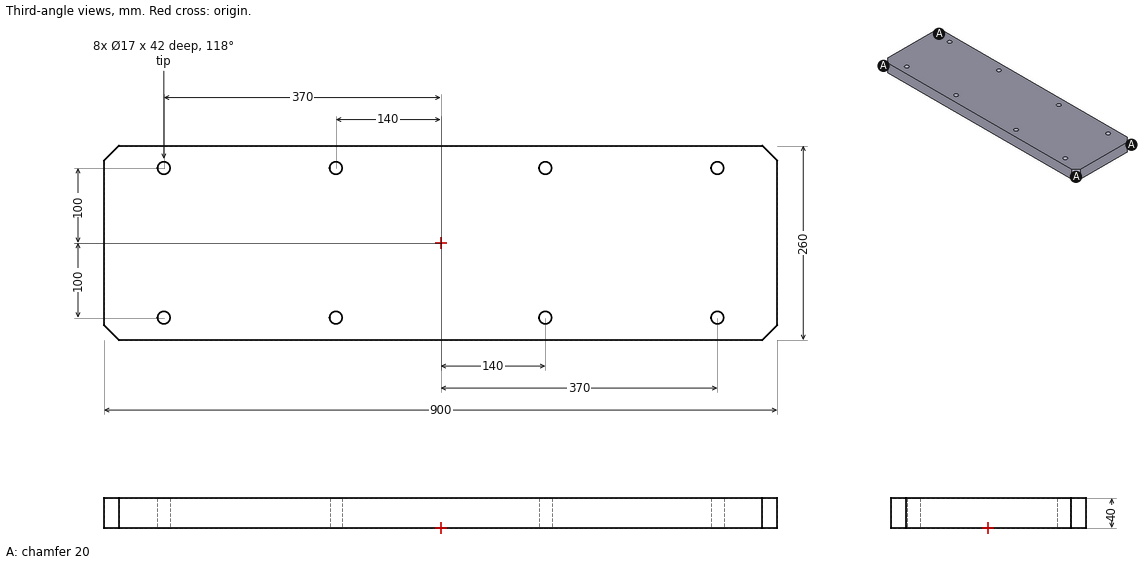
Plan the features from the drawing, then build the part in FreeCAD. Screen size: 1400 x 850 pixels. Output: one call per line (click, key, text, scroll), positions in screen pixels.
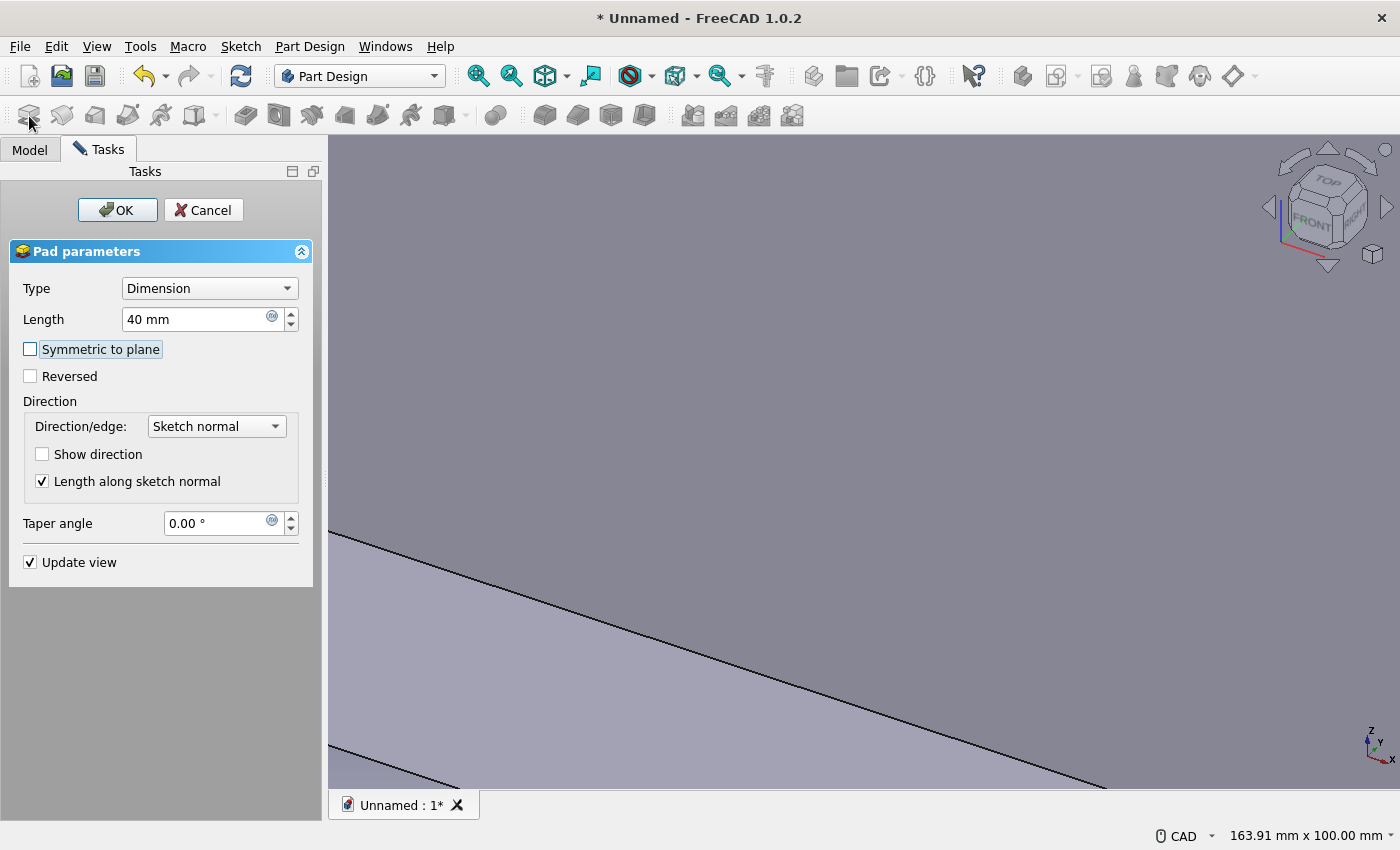
click(118, 210)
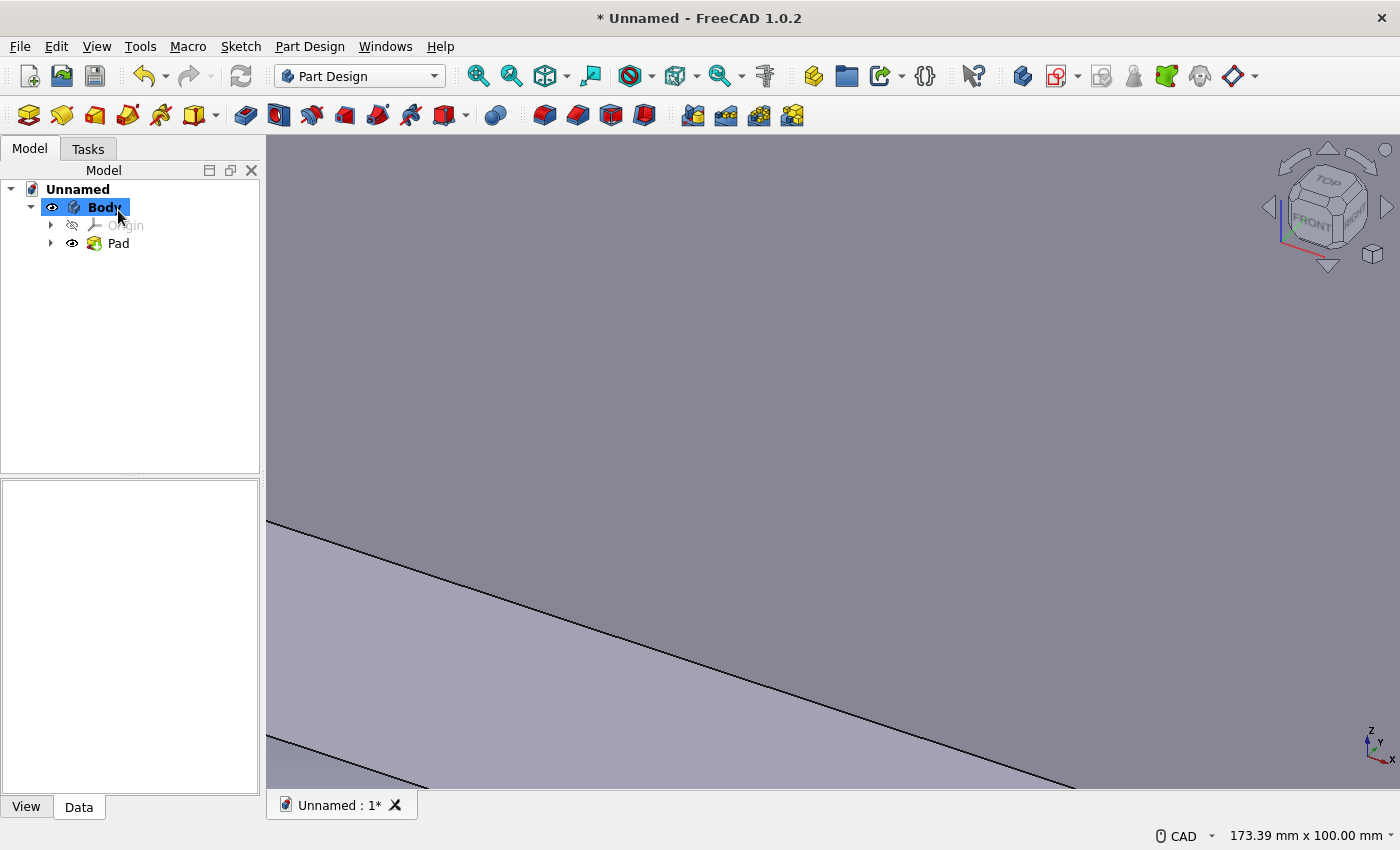
click(479, 76)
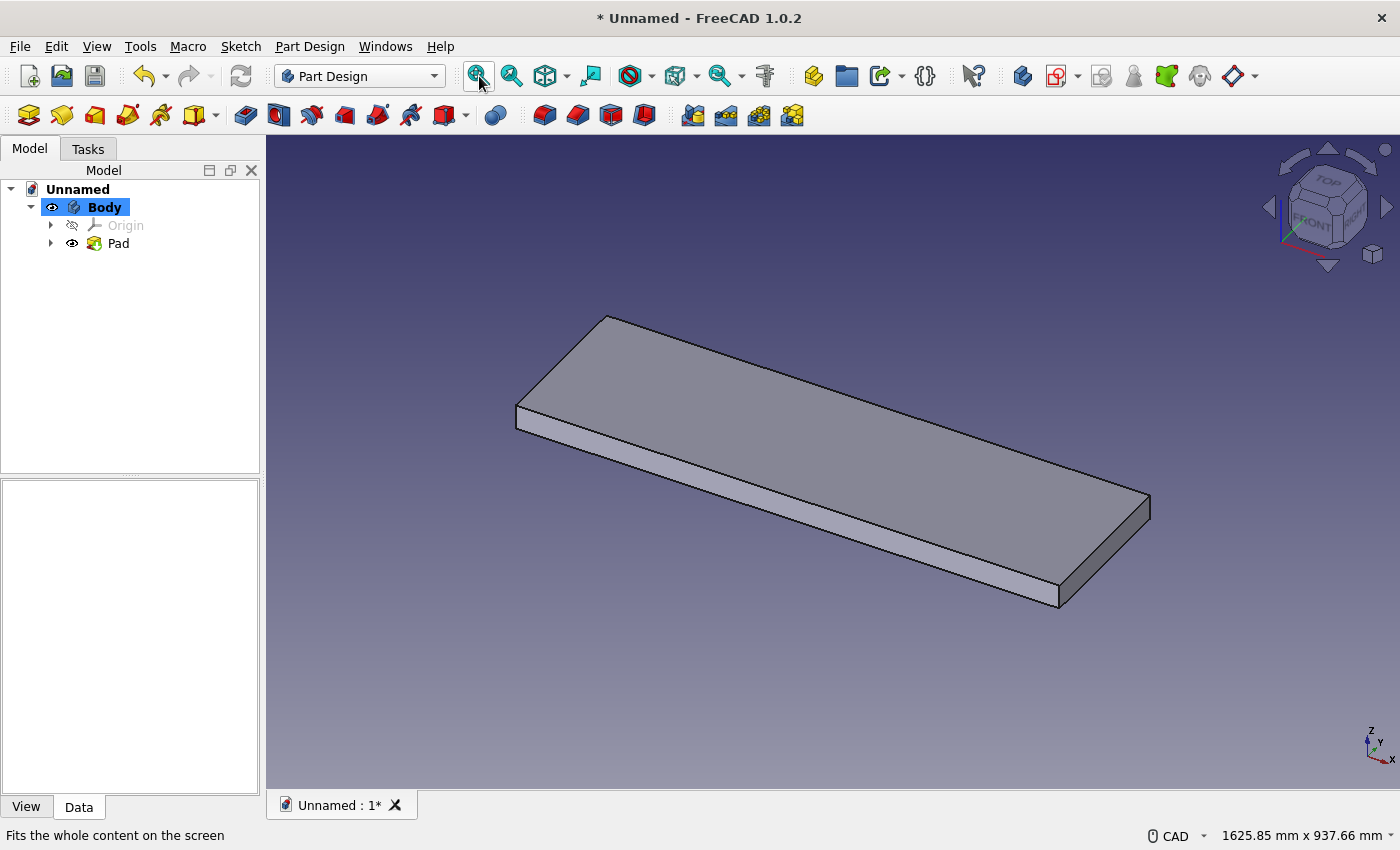
click(988, 501)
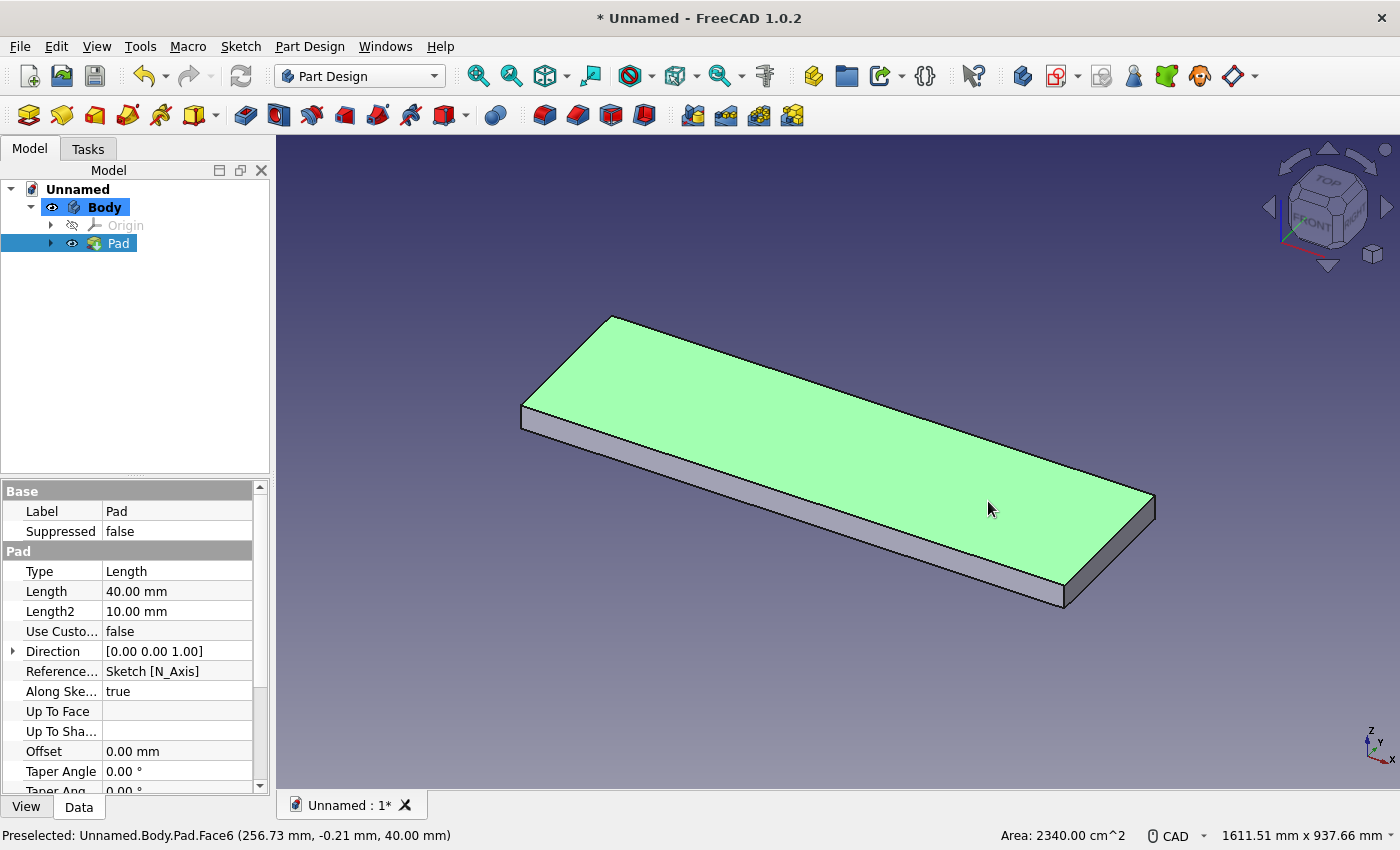
click(1056, 76)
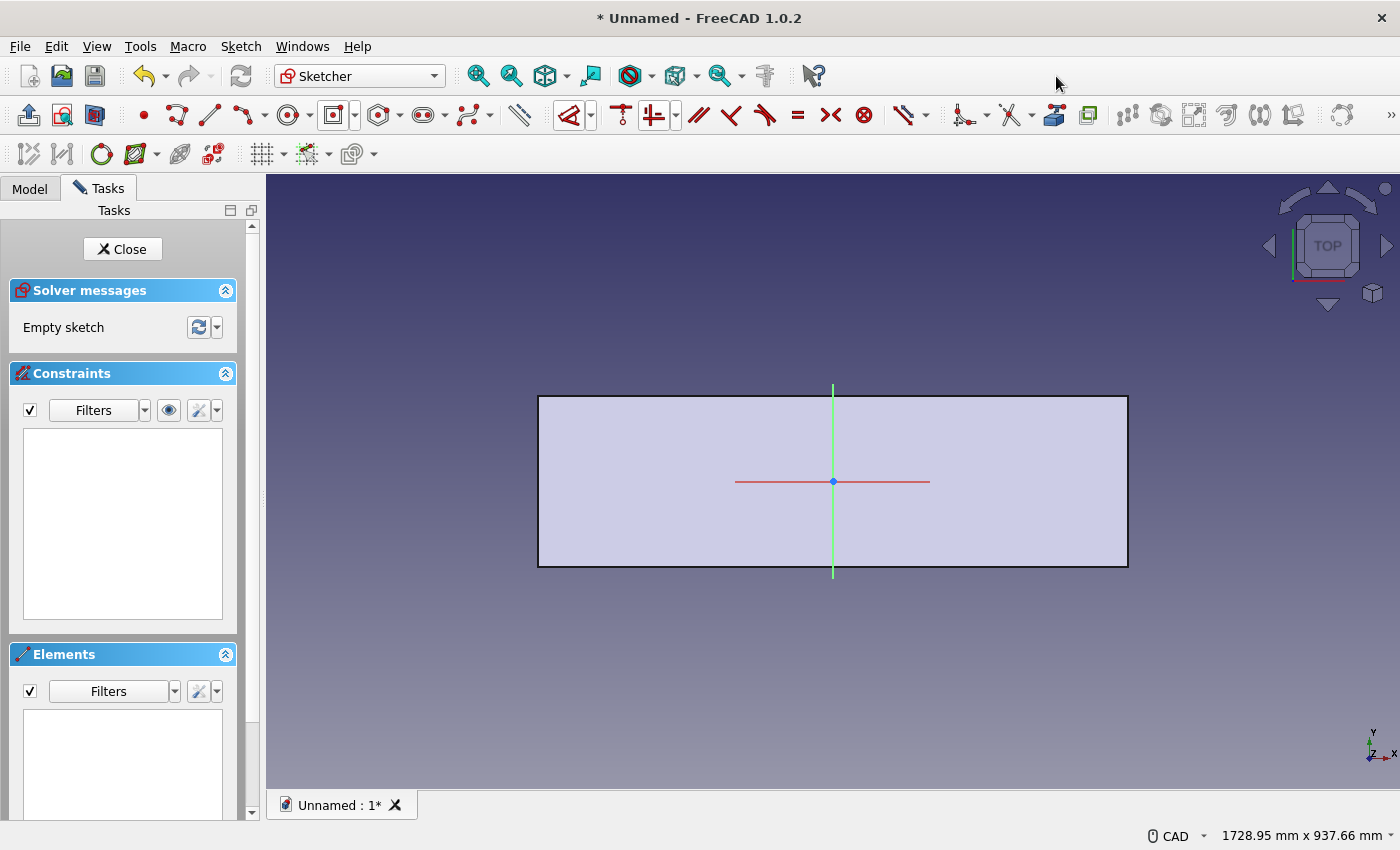
click(288, 116)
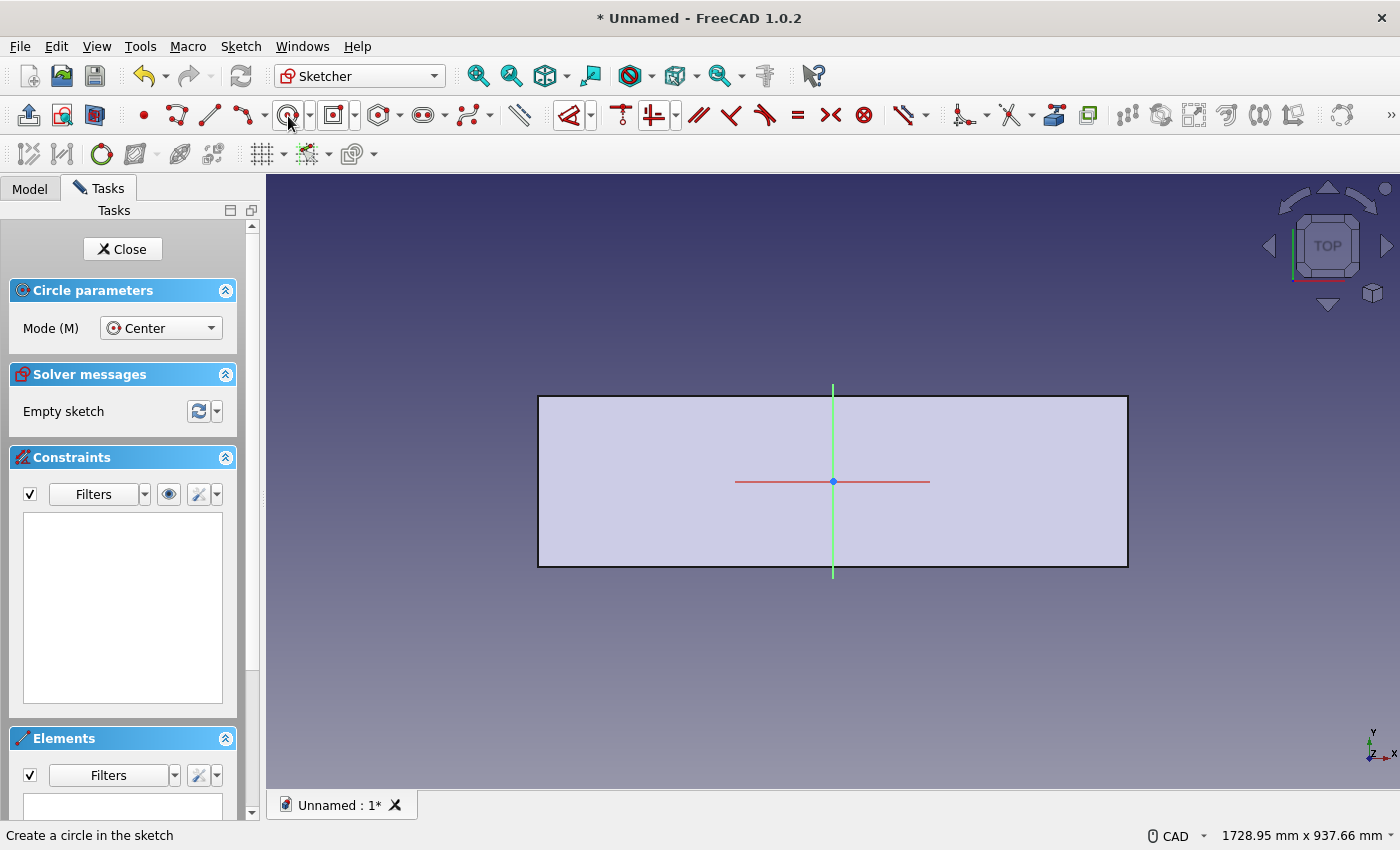
scroll(590, 416, up, 8)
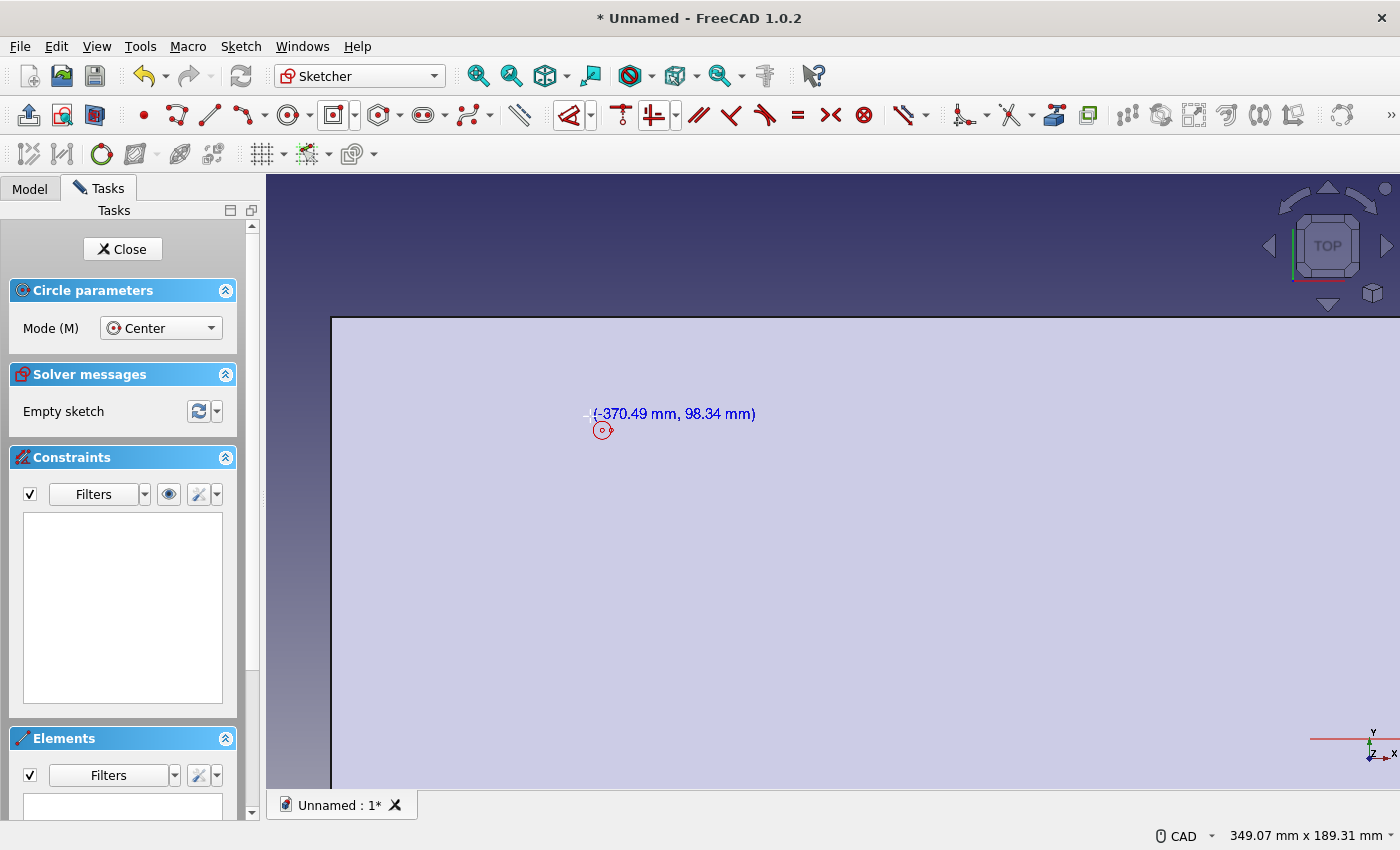
scroll(428, 397, down, 7)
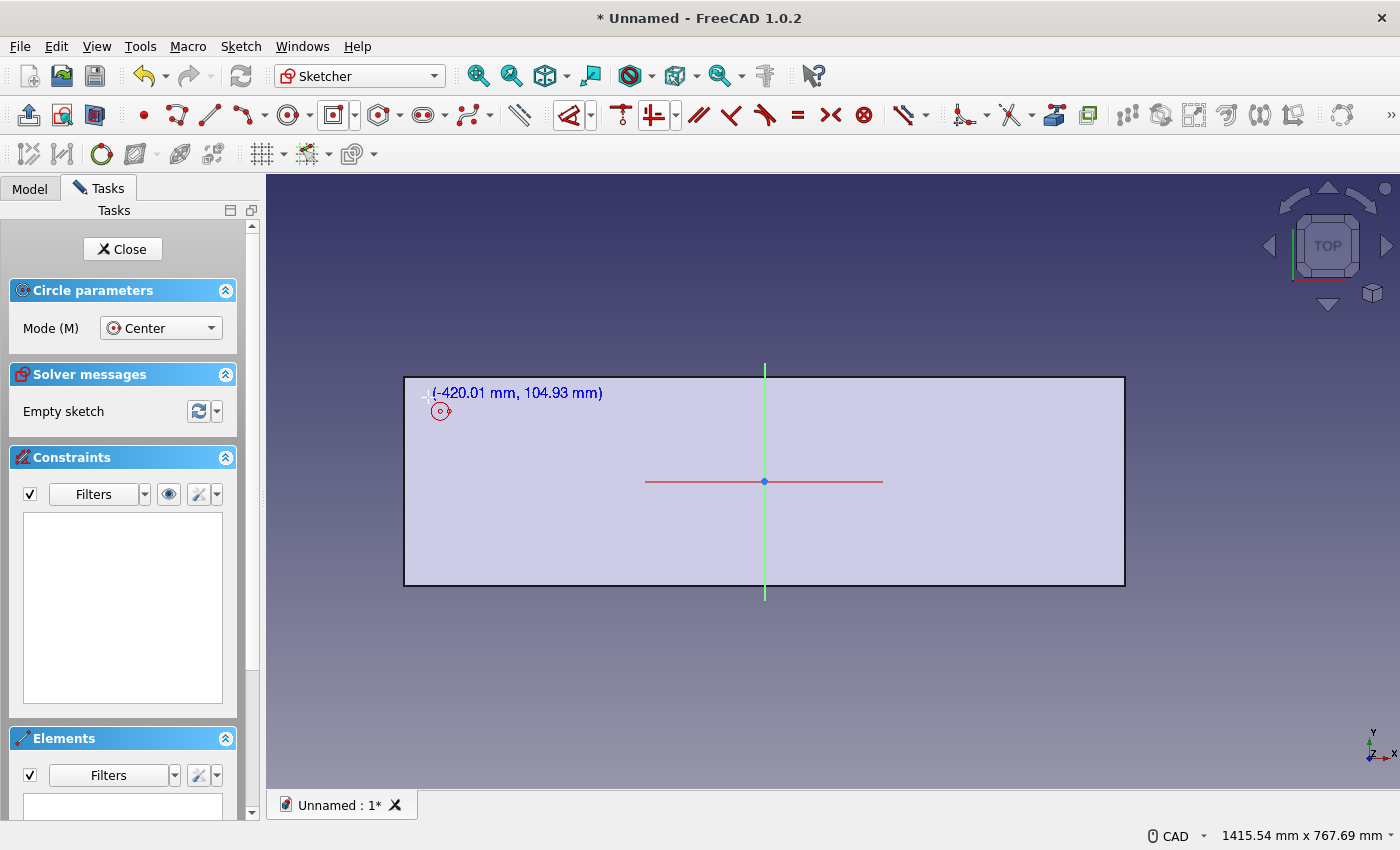
click(468, 401)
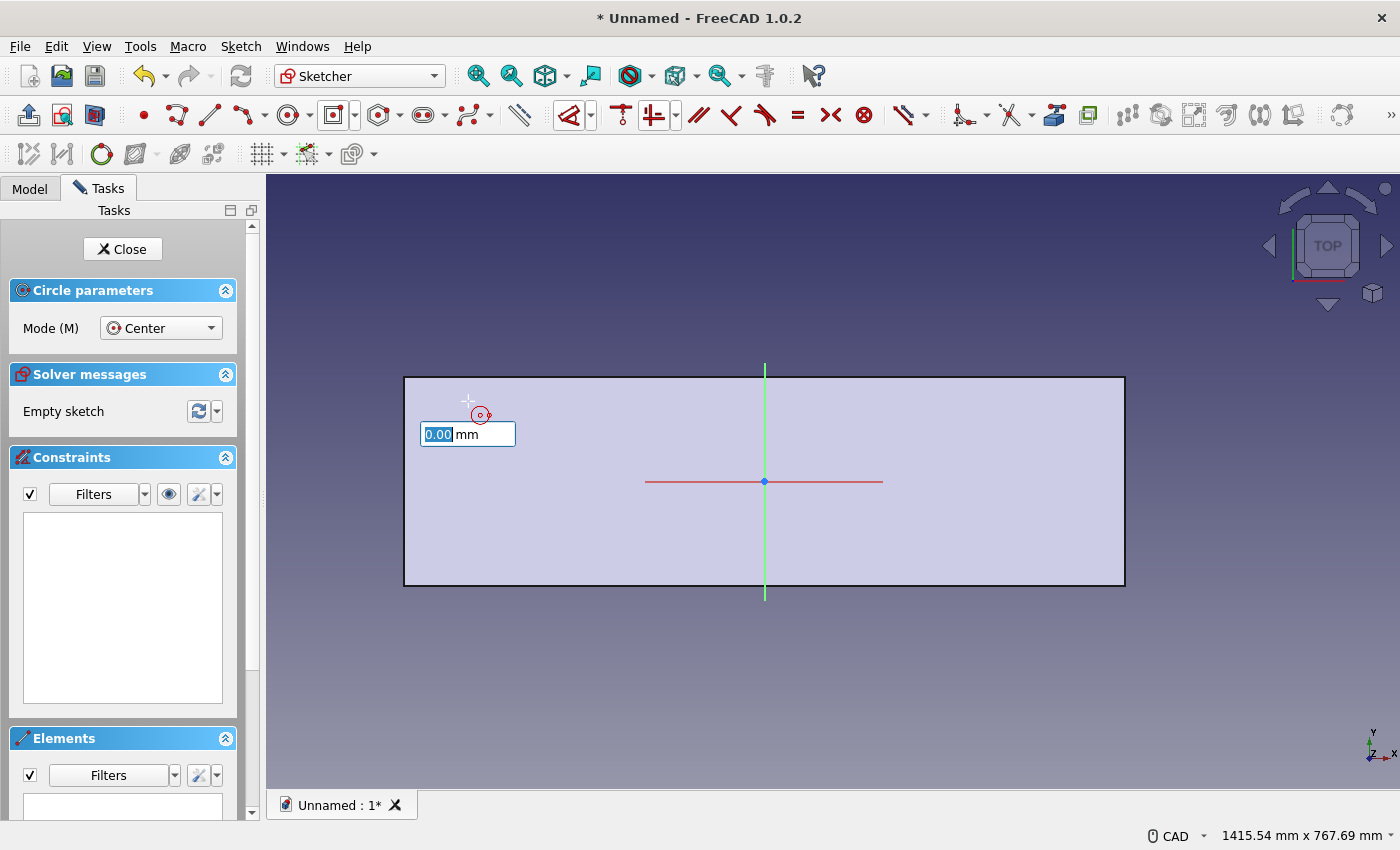
scroll(473, 397, up, 5)